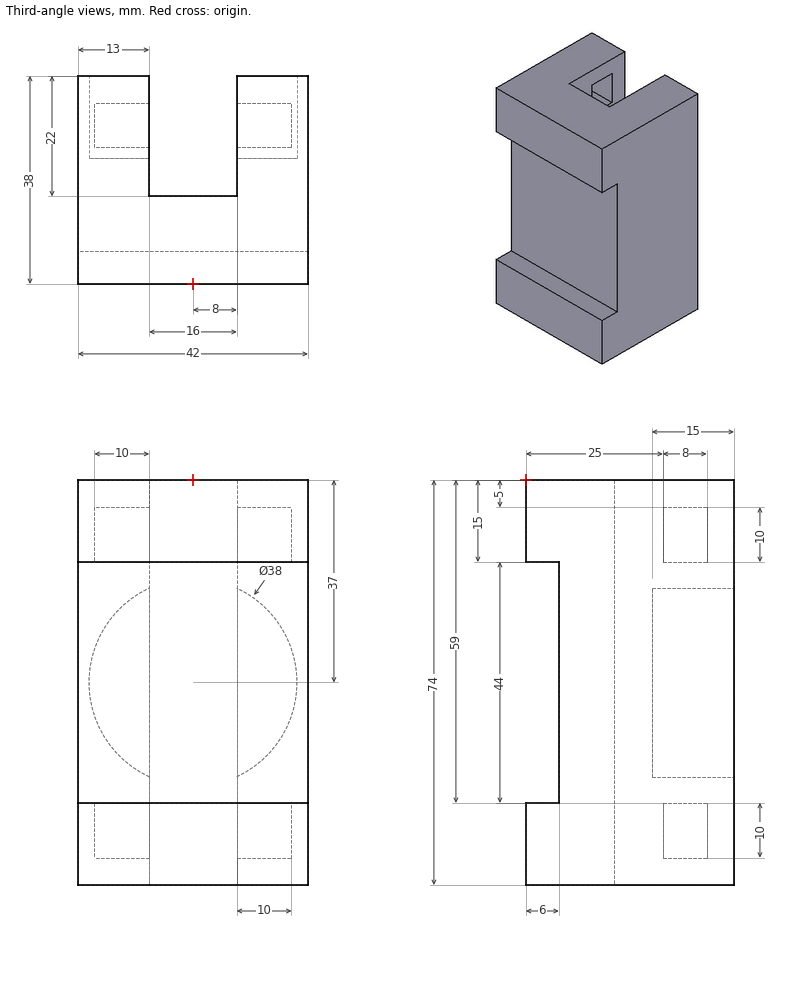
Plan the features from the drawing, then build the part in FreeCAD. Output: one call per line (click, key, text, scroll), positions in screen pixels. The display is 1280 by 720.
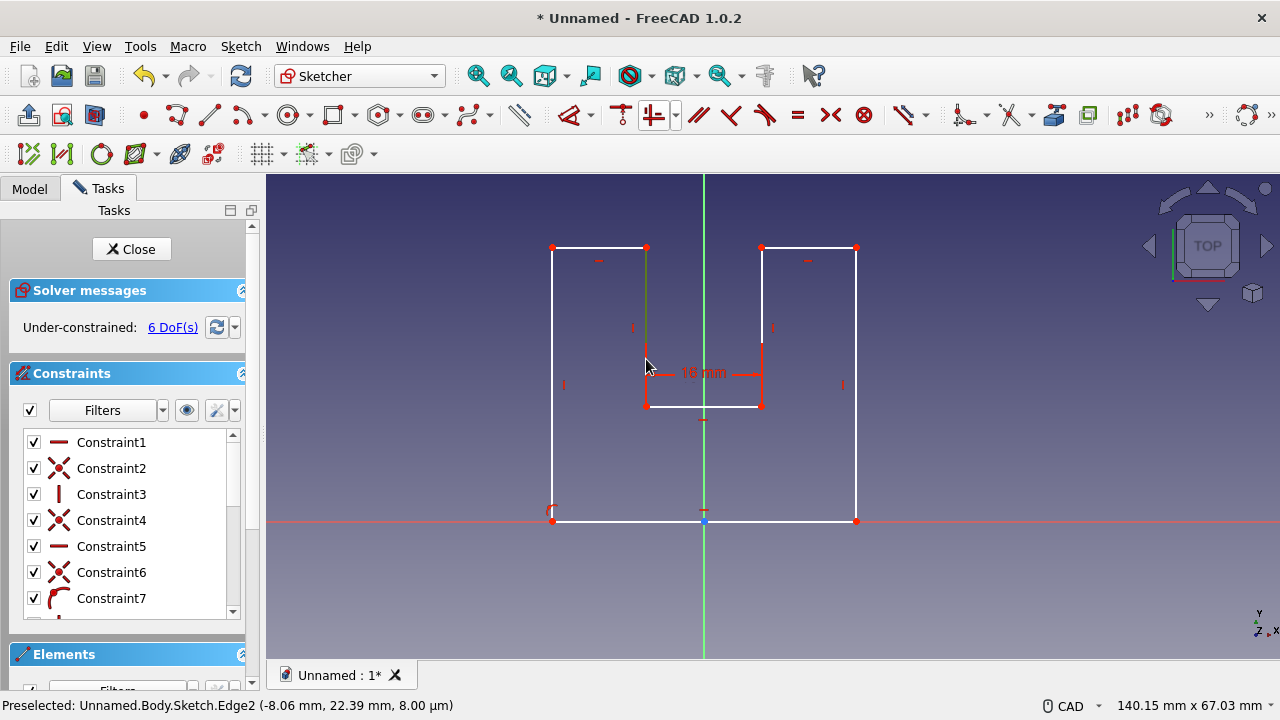
key(i)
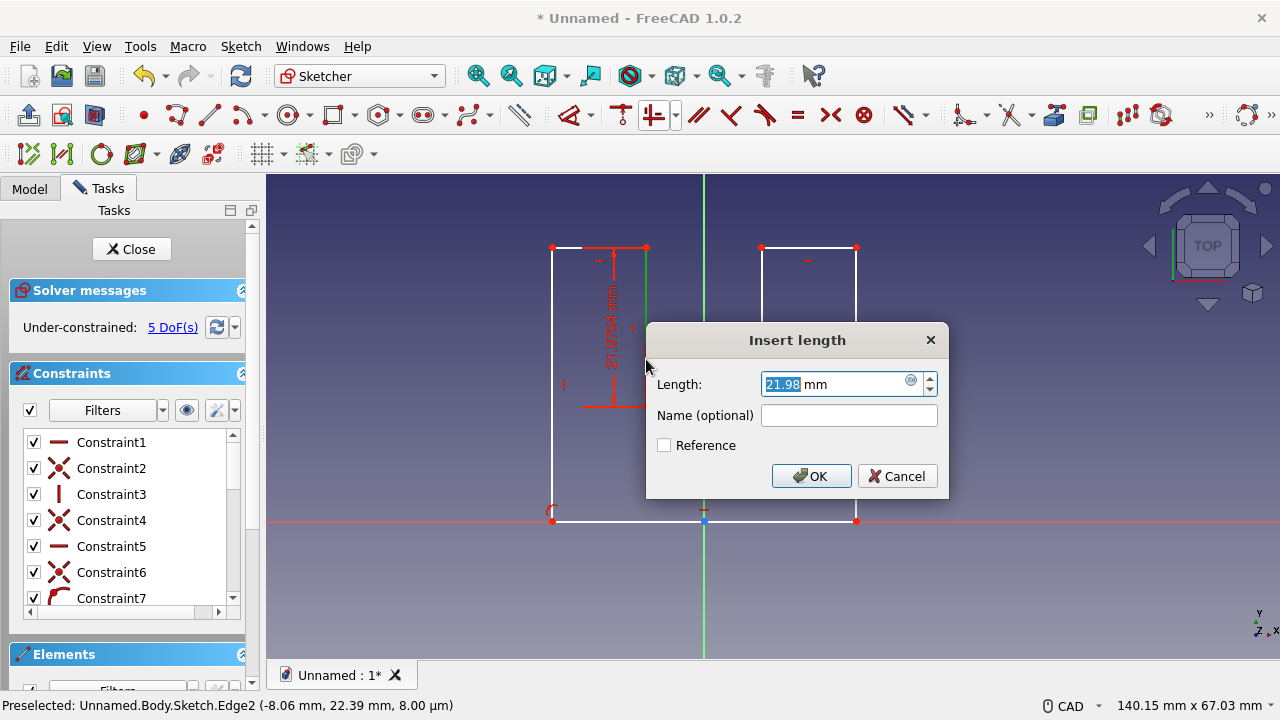
text(22)
key(Return)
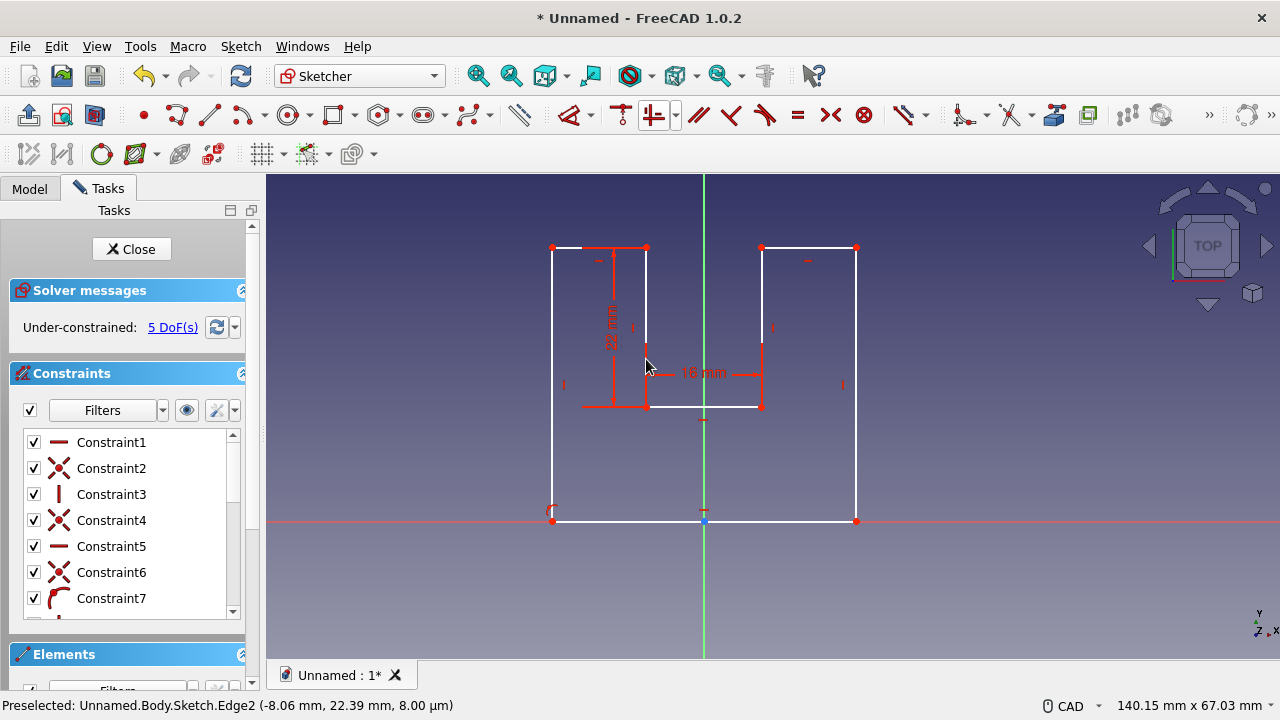
click(618, 248)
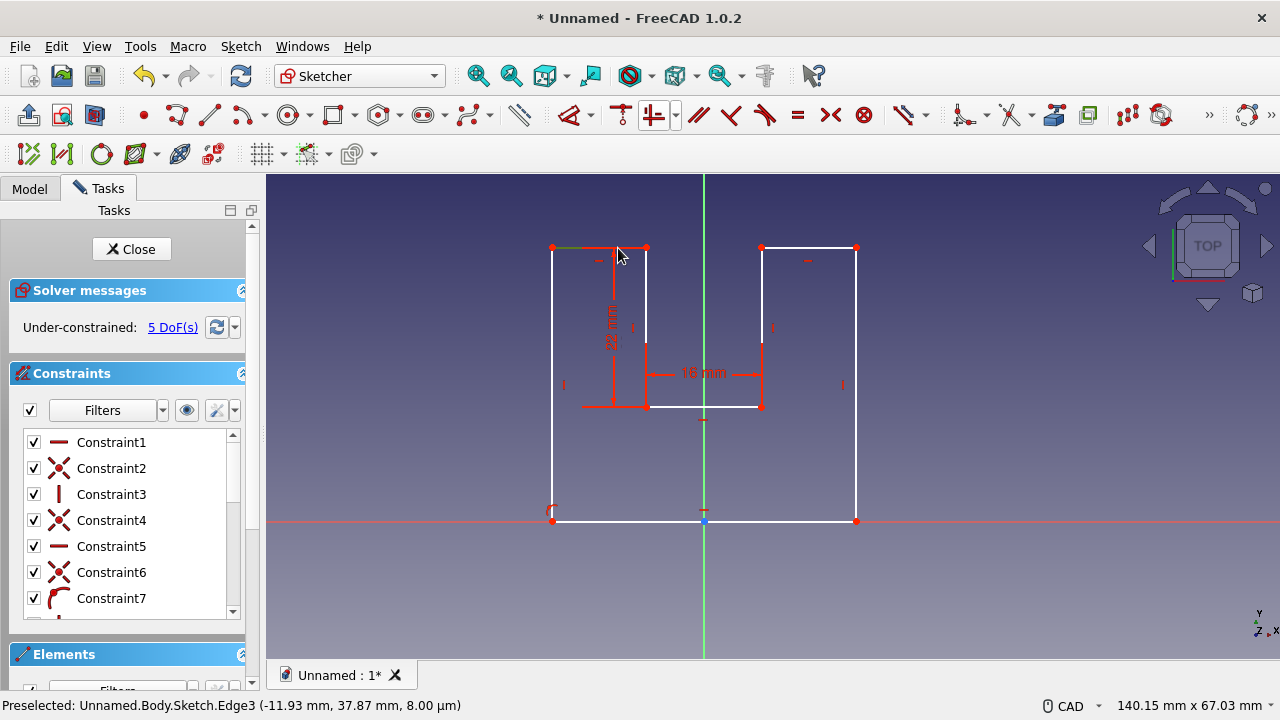
click(590, 116)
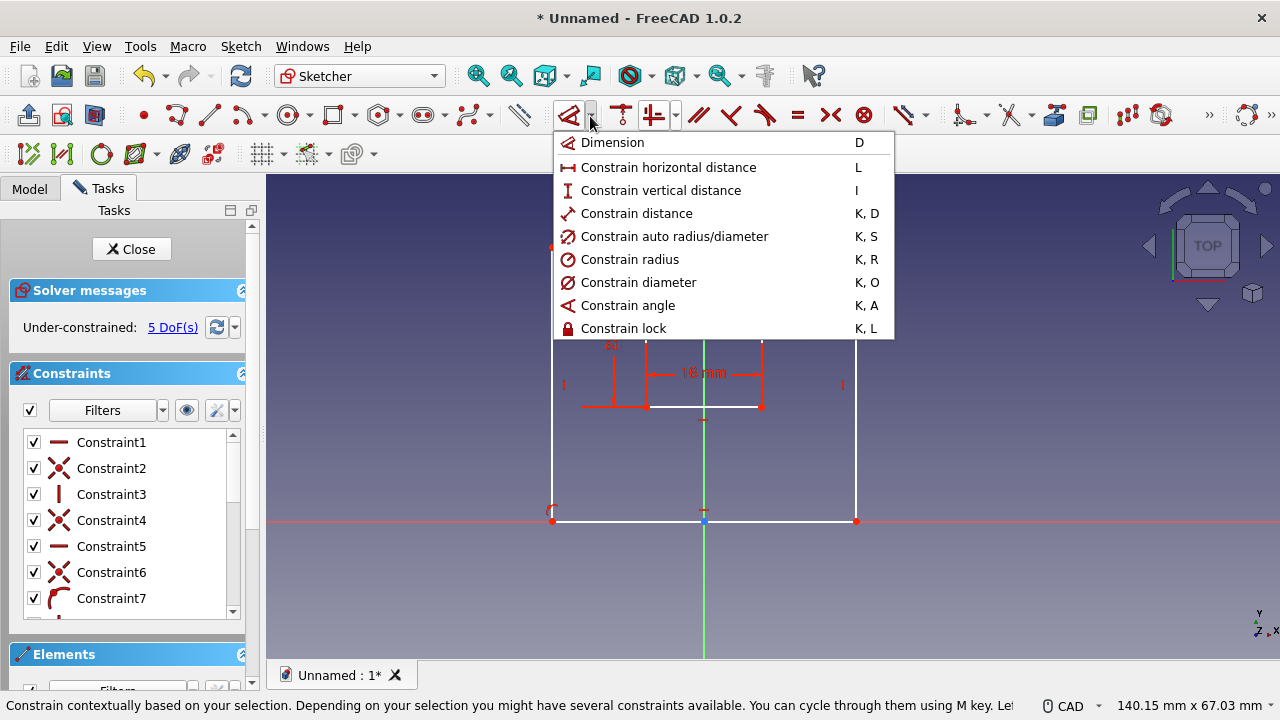
click(724, 168)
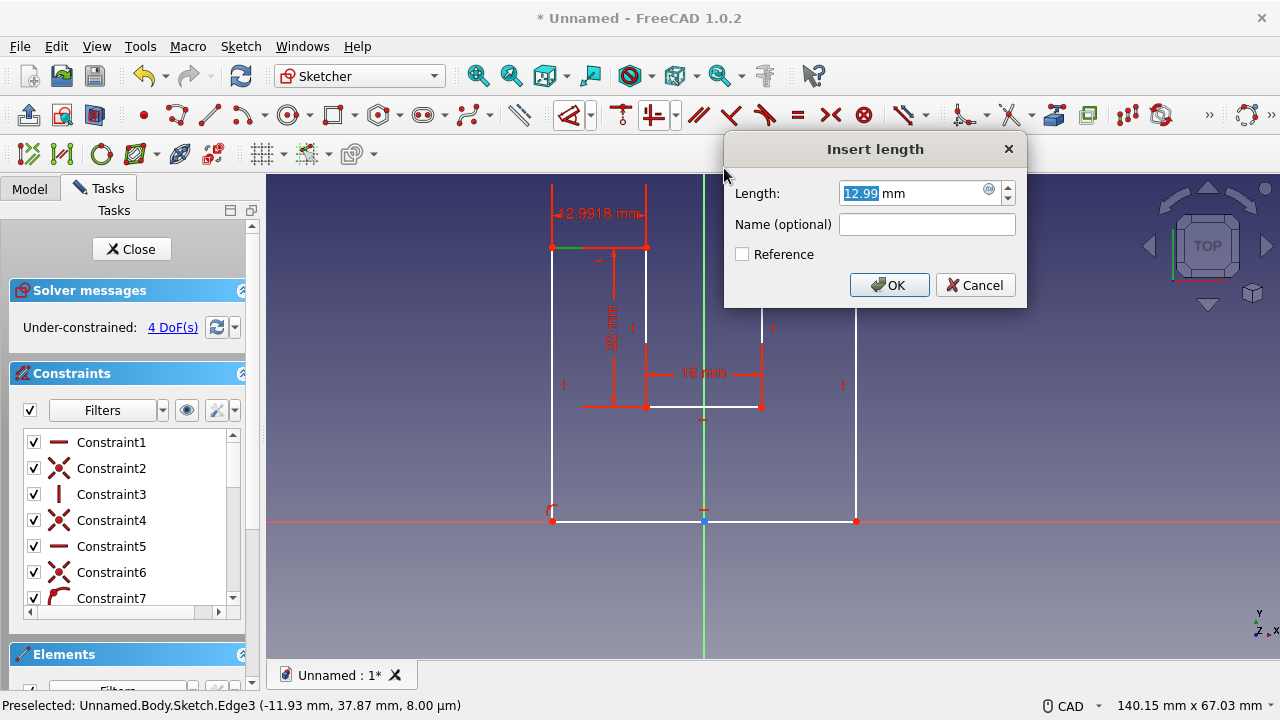
text(13)
key(Return)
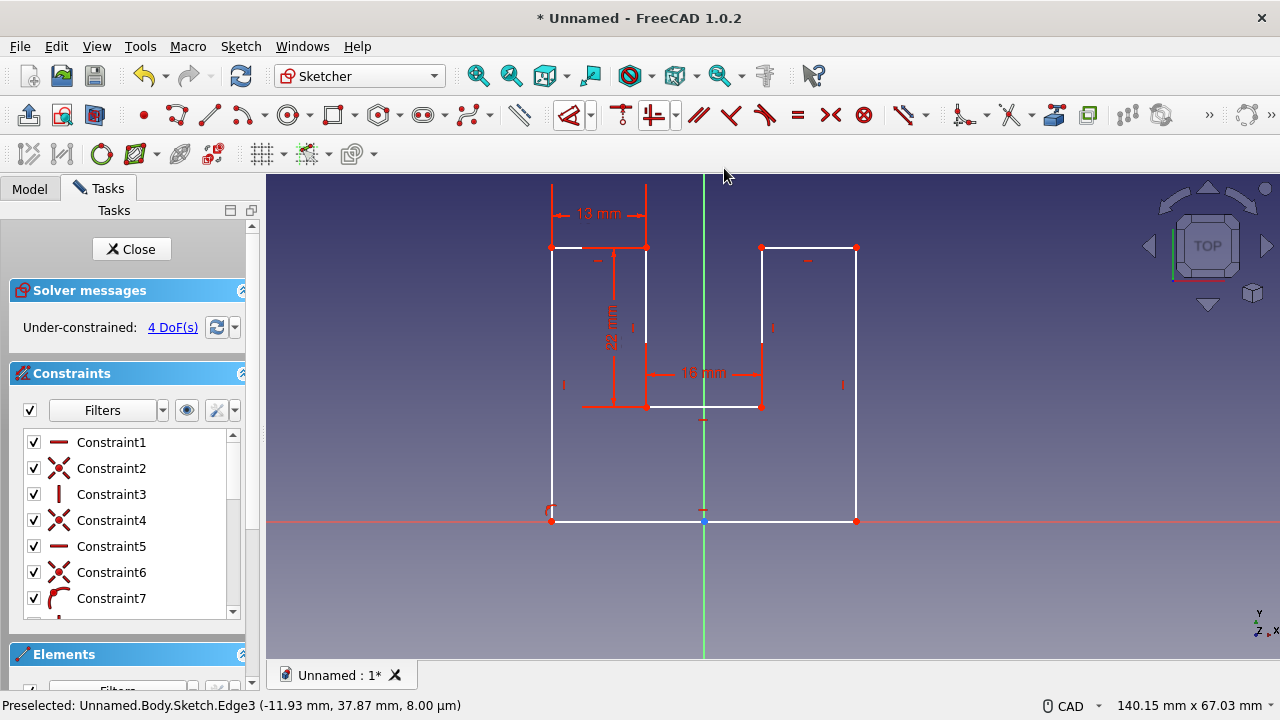
click(552, 330)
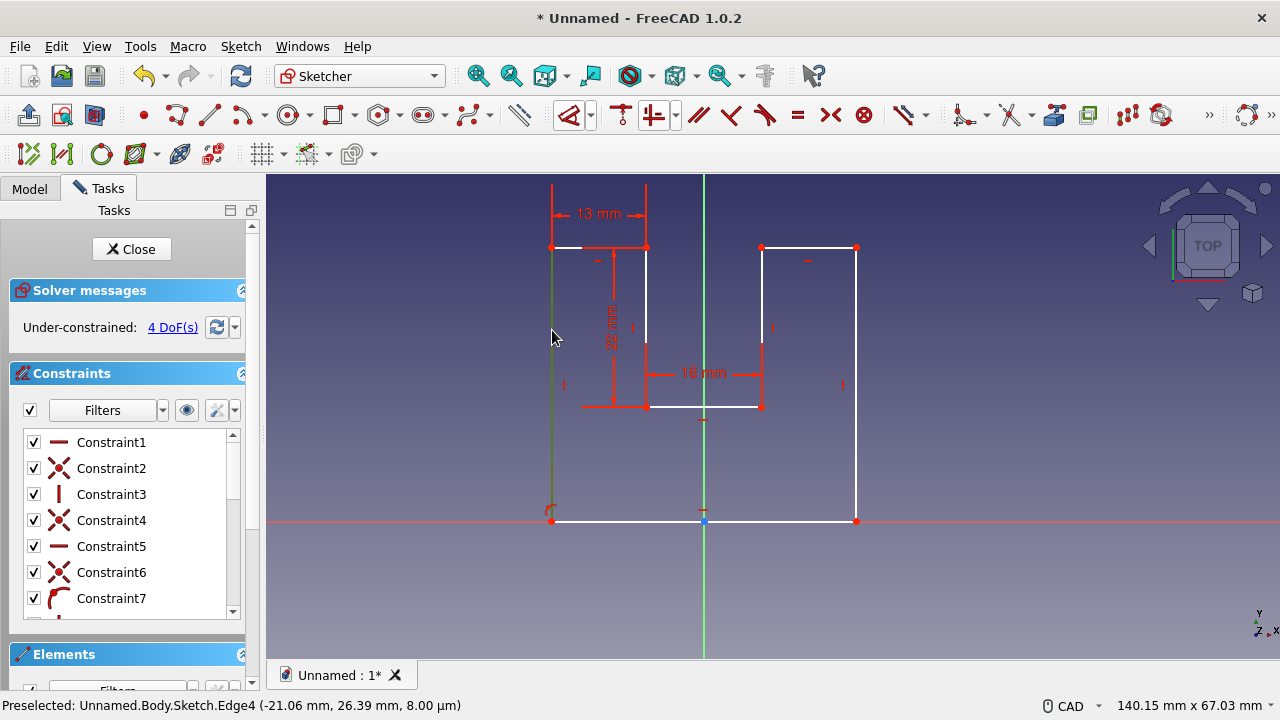
click(590, 116)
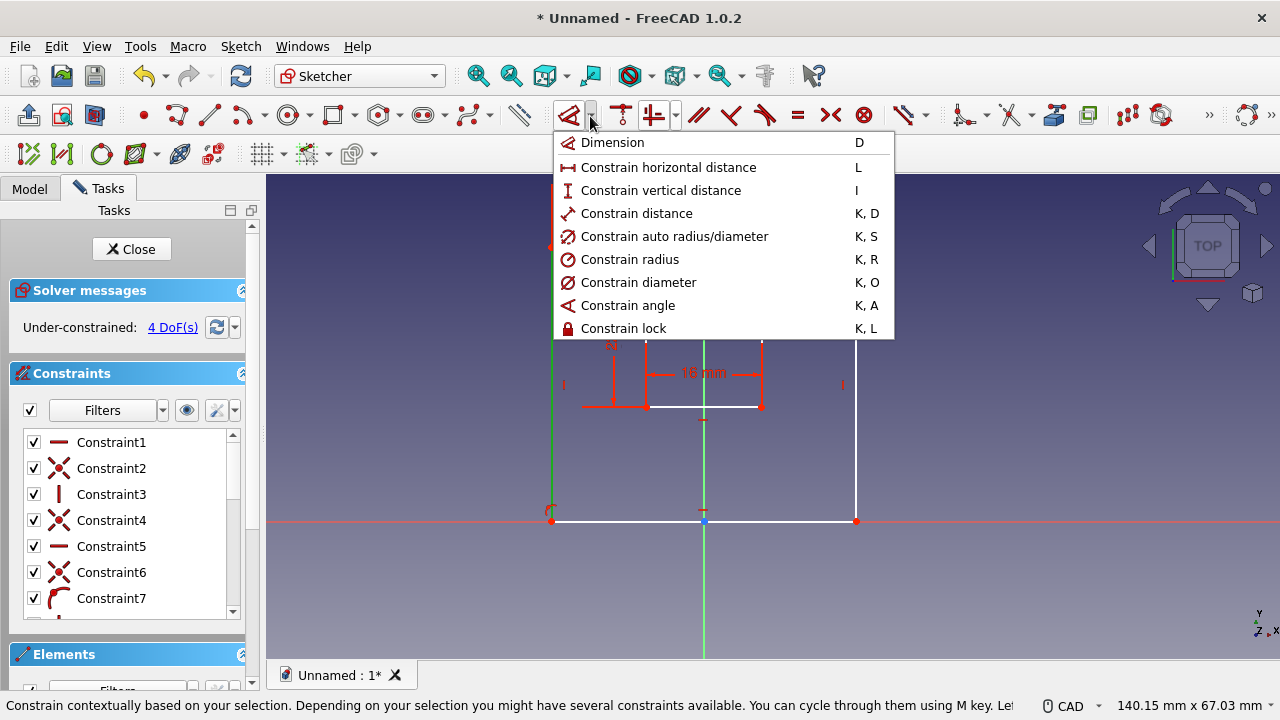
click(724, 190)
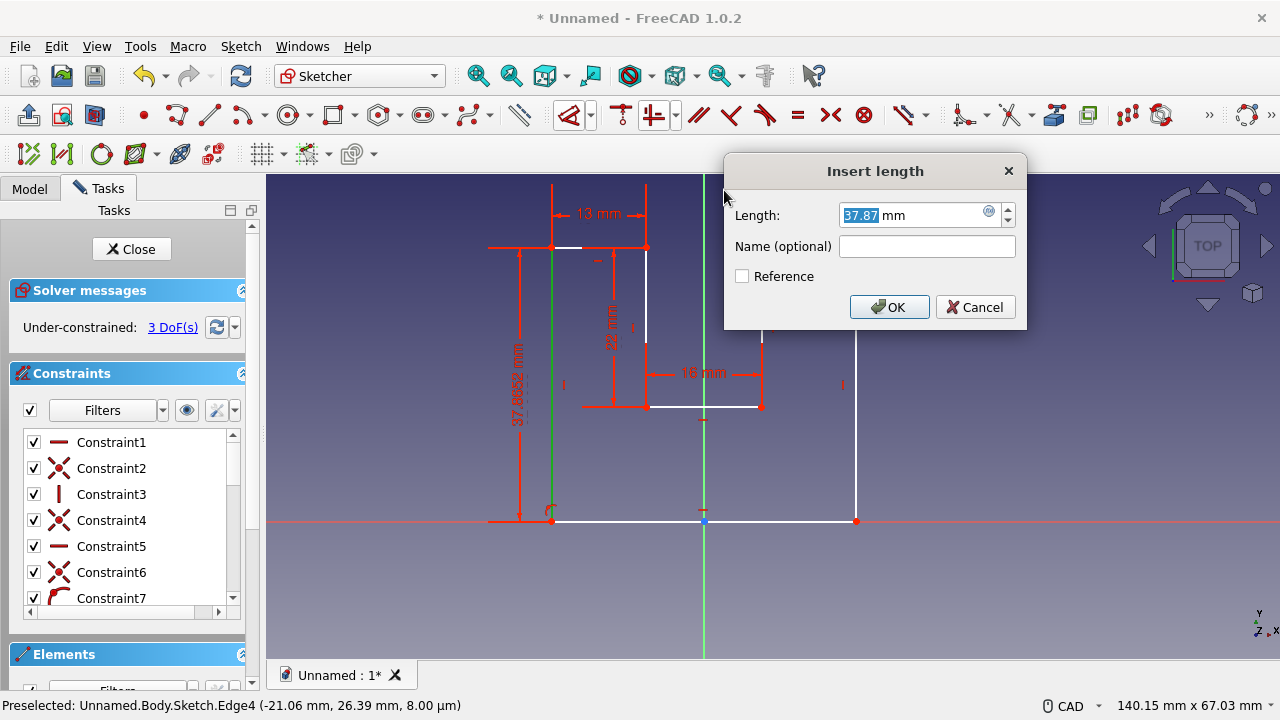
text(38)
key(Return)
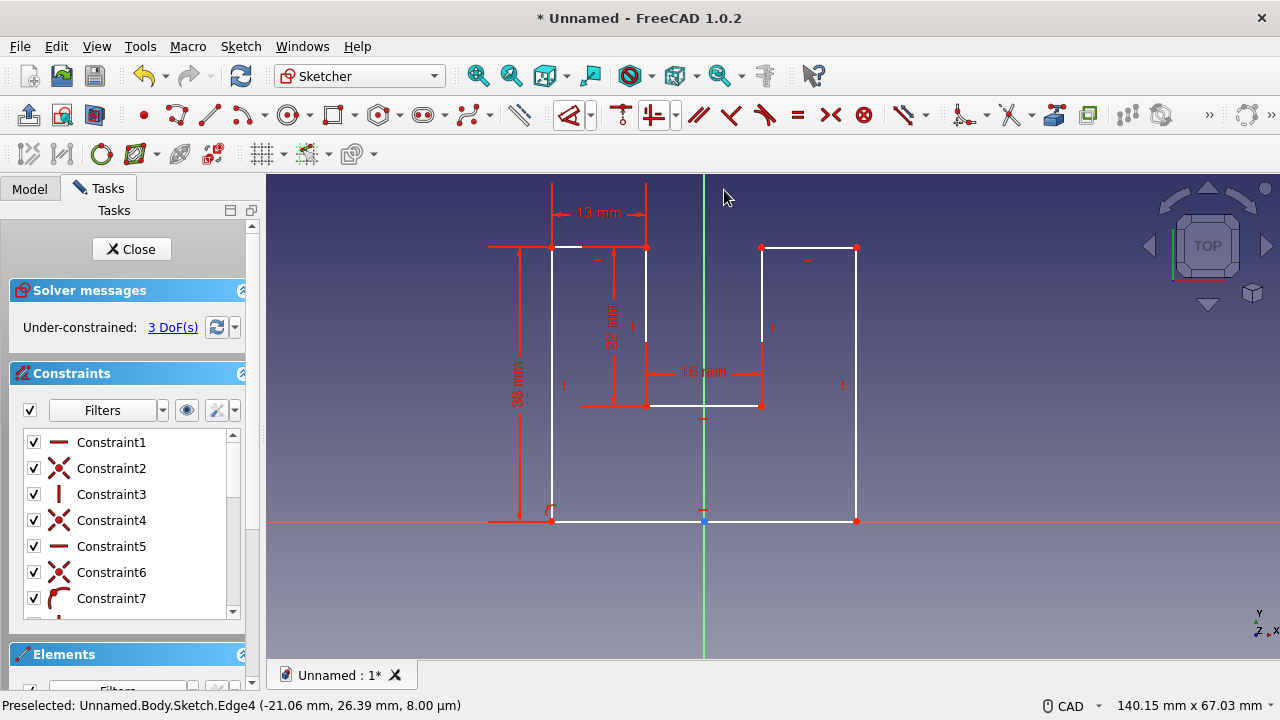
click(643, 522)